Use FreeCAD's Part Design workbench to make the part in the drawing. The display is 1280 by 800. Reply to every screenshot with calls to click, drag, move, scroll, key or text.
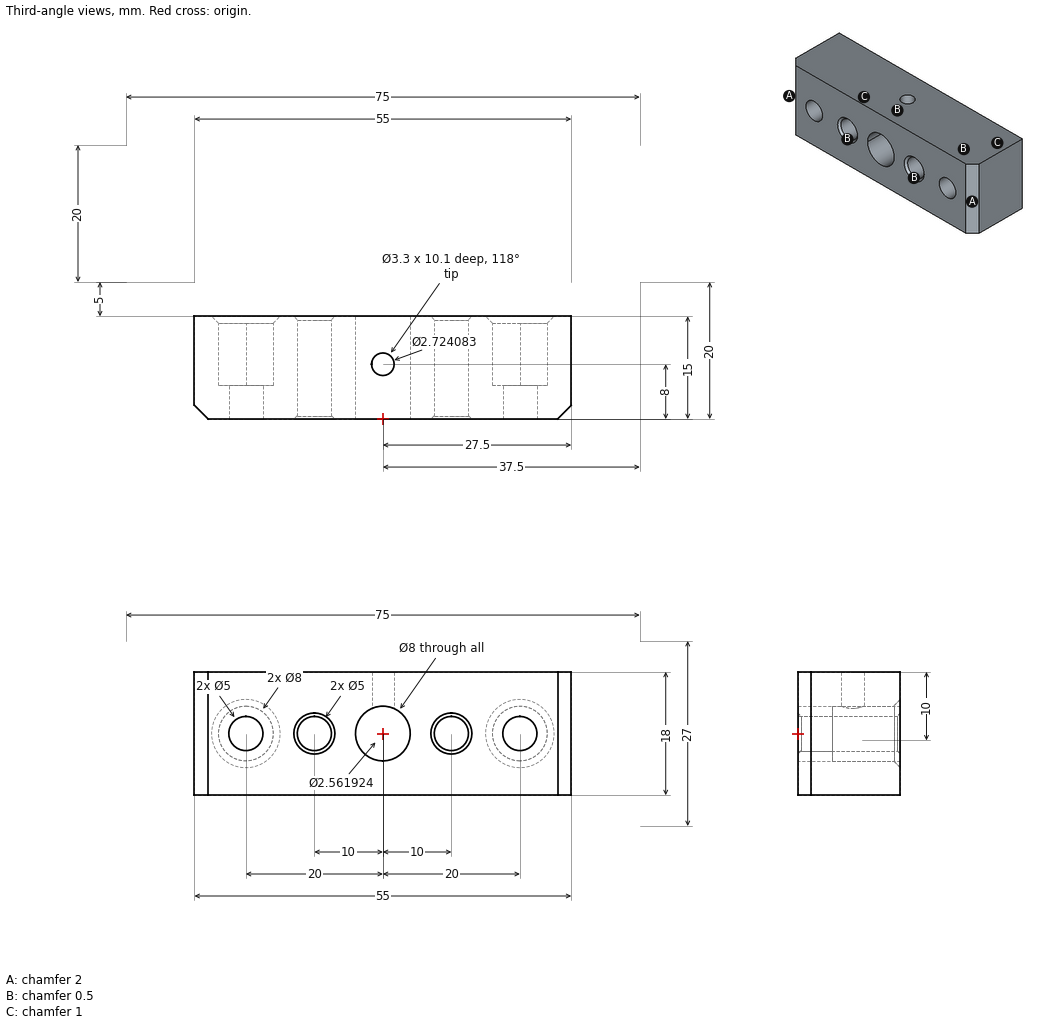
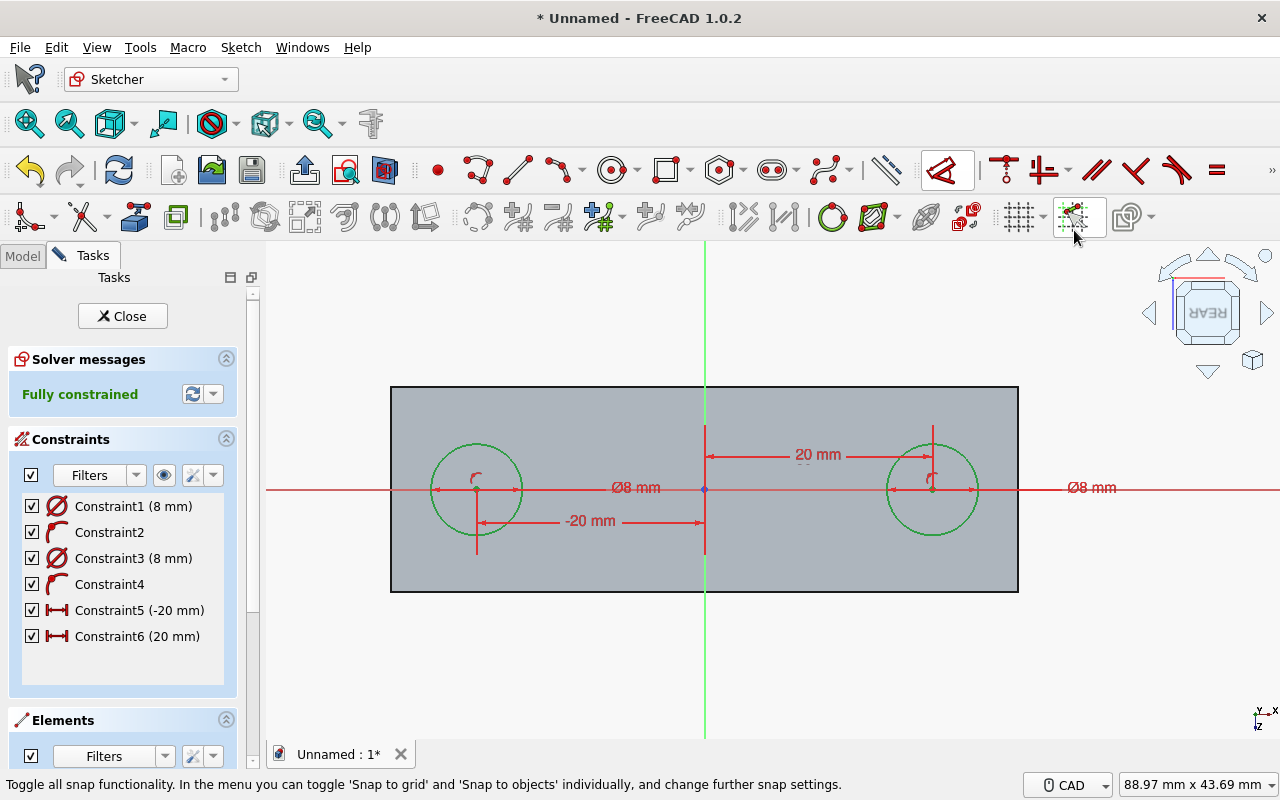
click(123, 316)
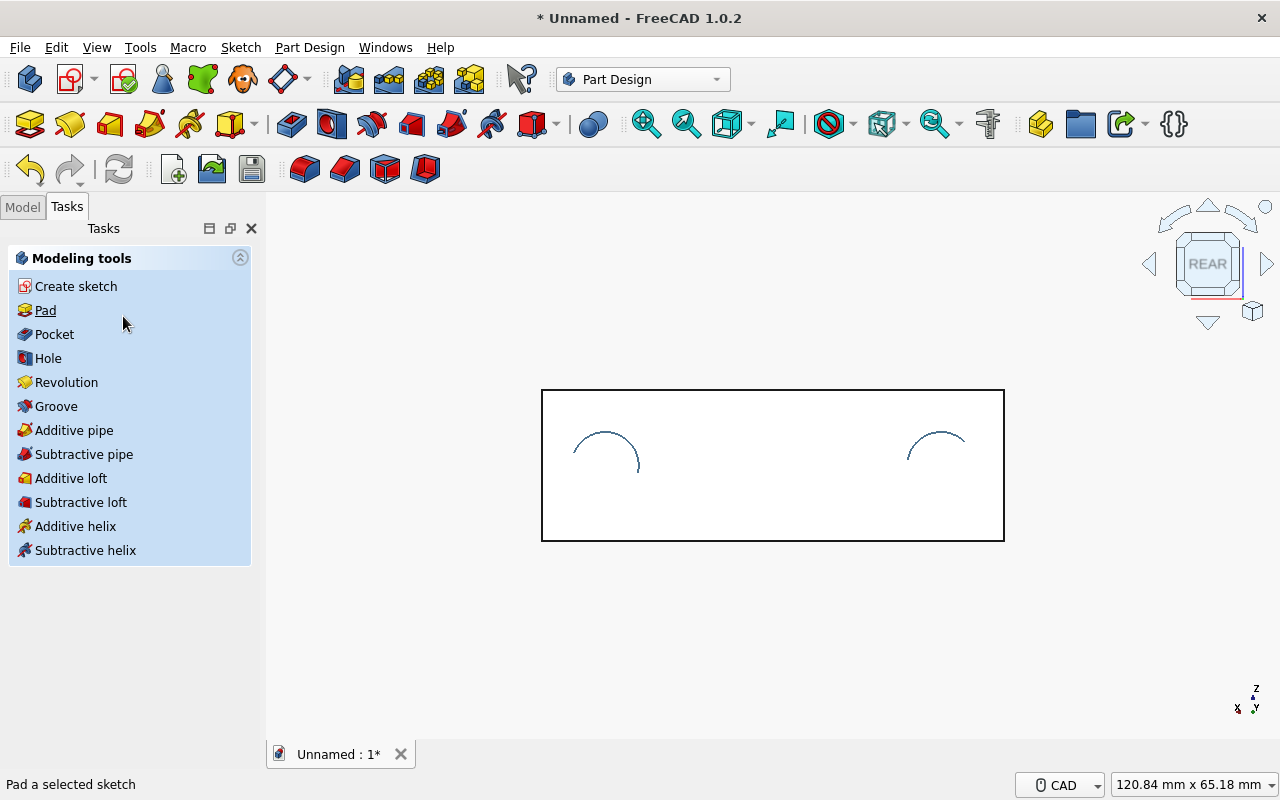
click(292, 124)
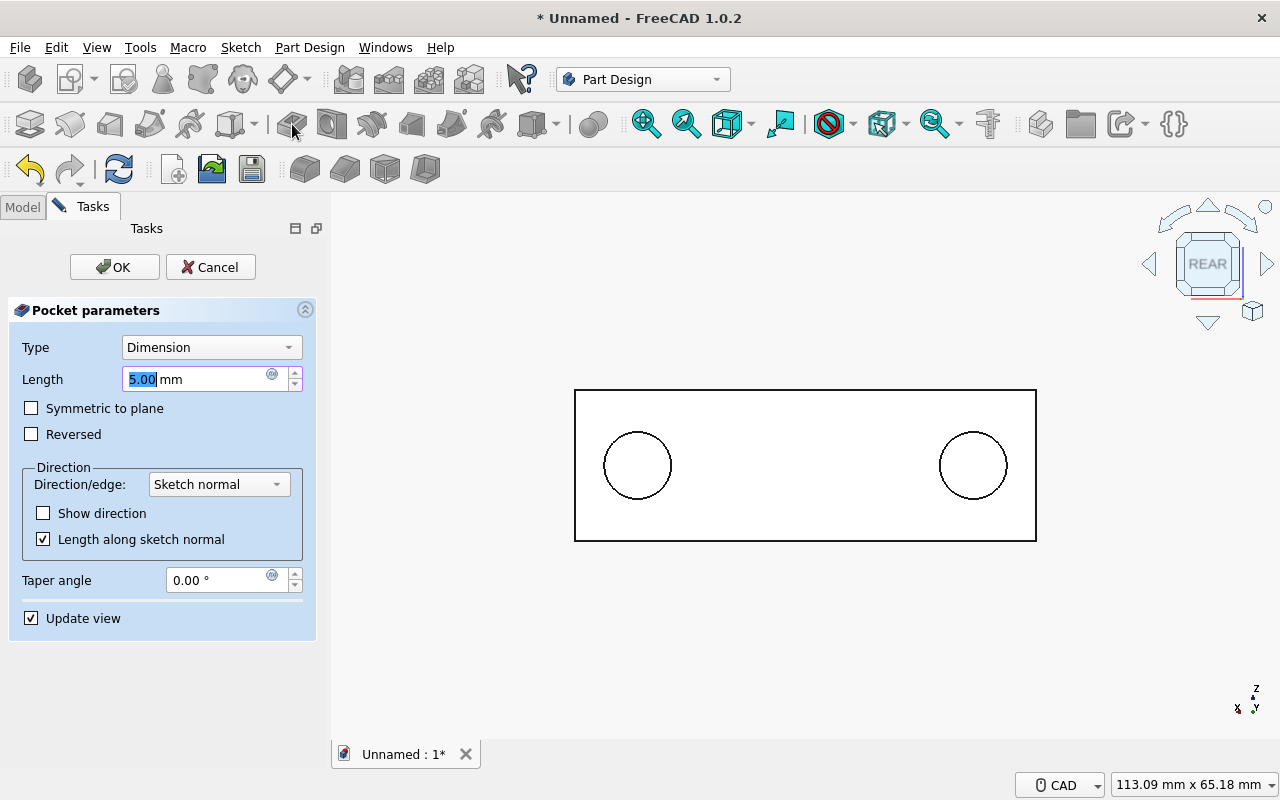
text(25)
key(Tab)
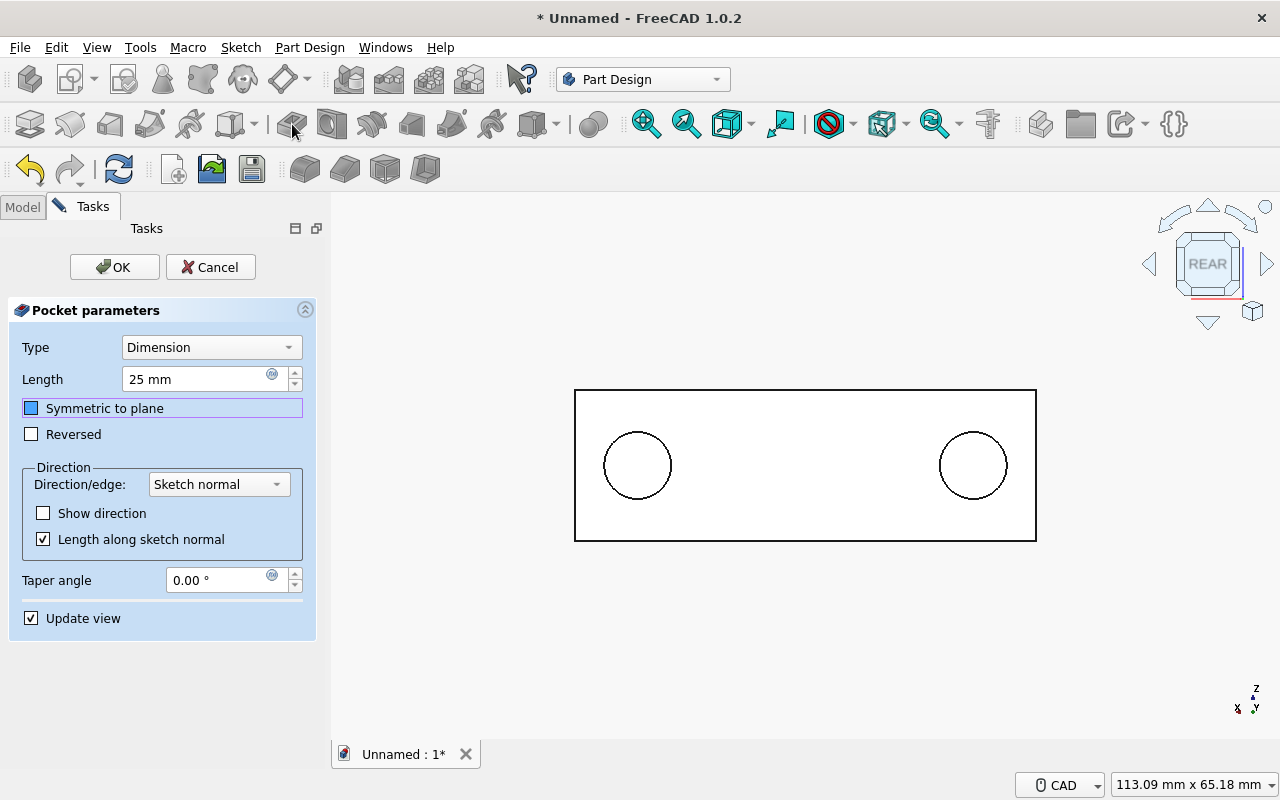
click(115, 267)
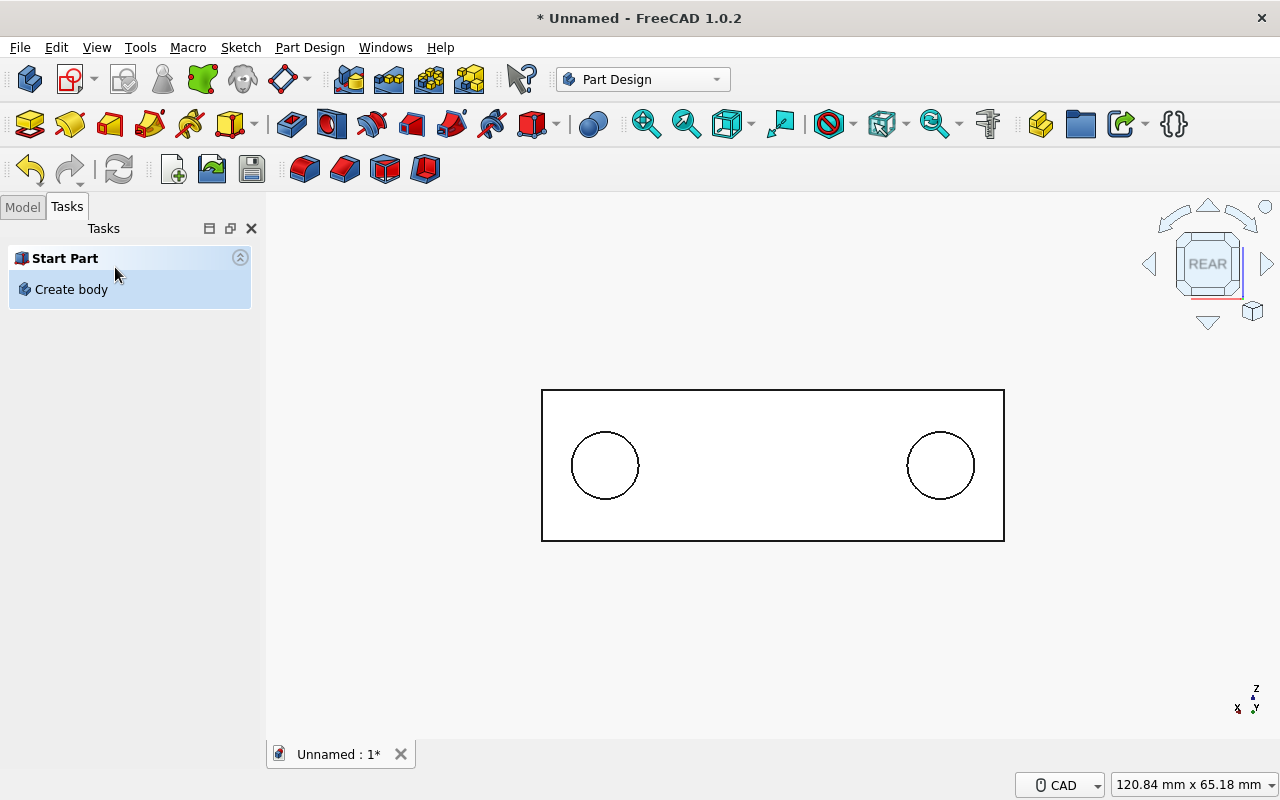
click(773, 465)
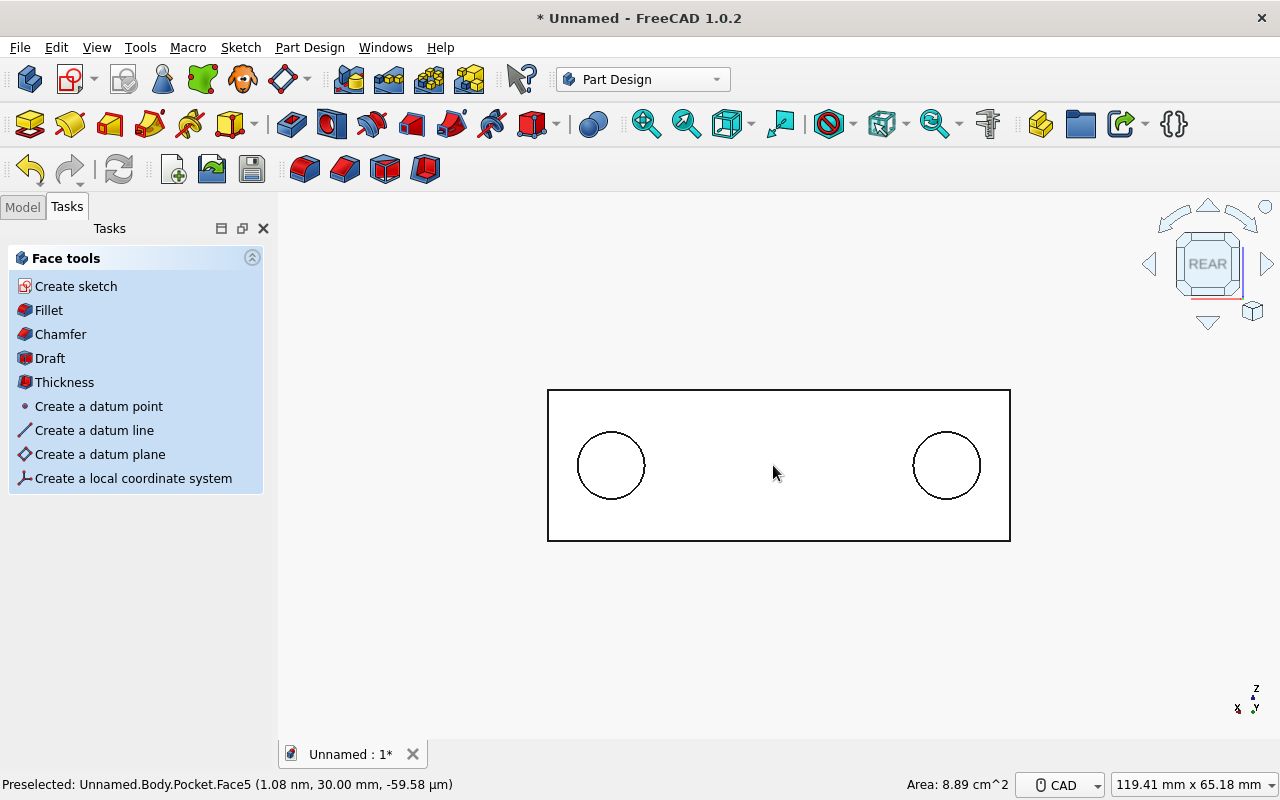
click(70, 80)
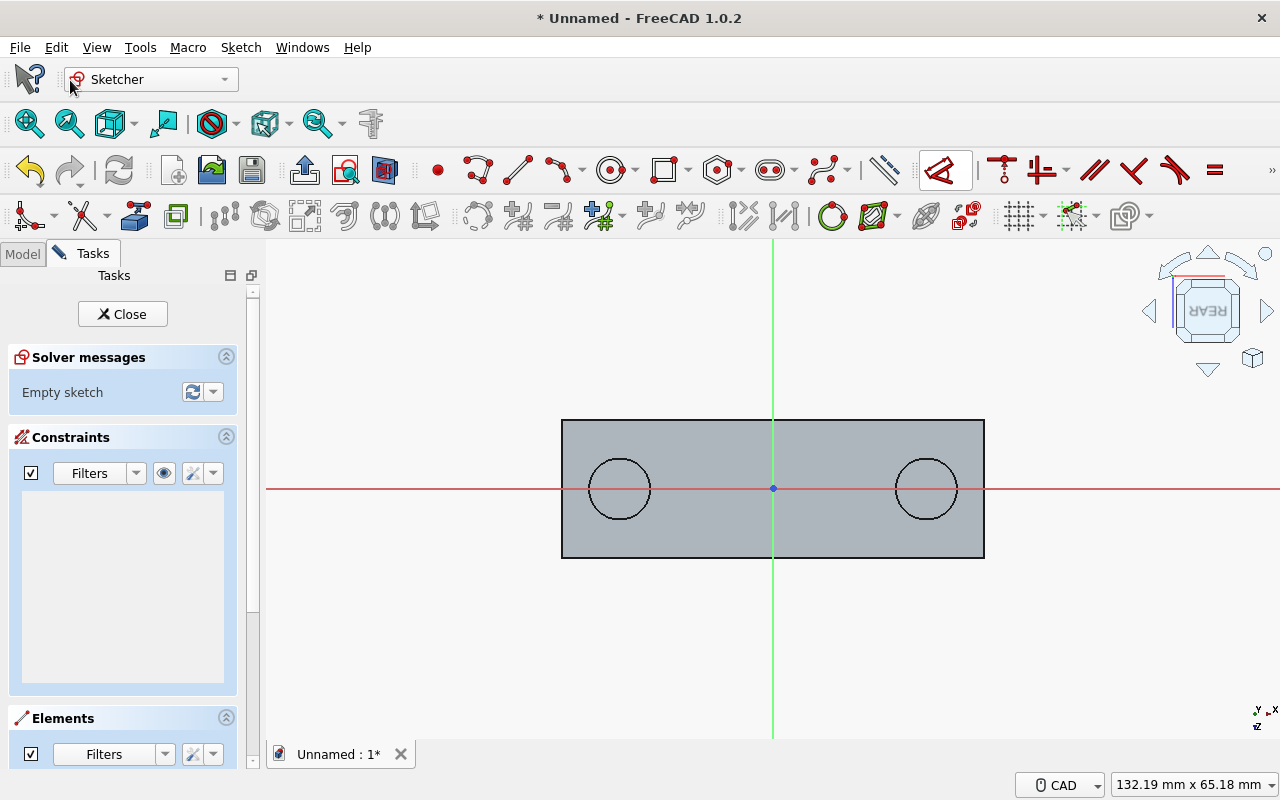
scroll(856, 489, up, 3)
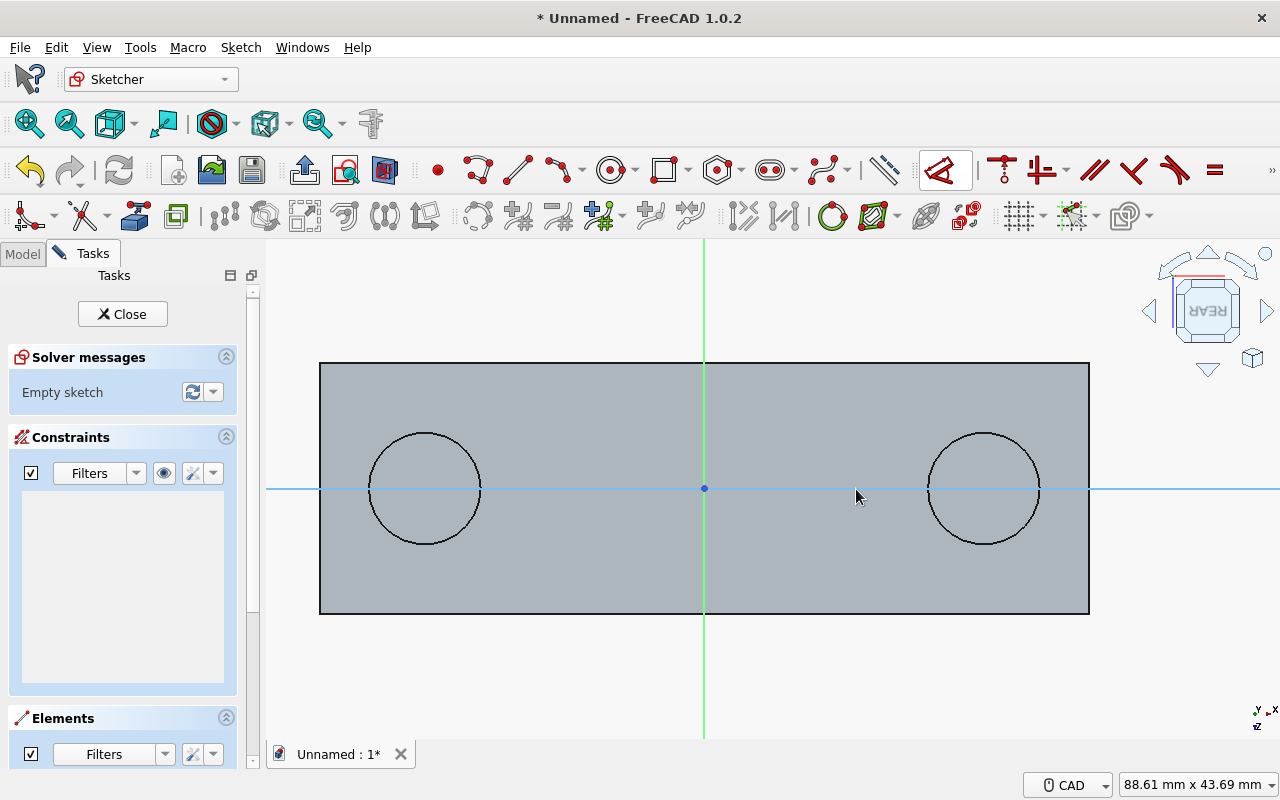
click(612, 170)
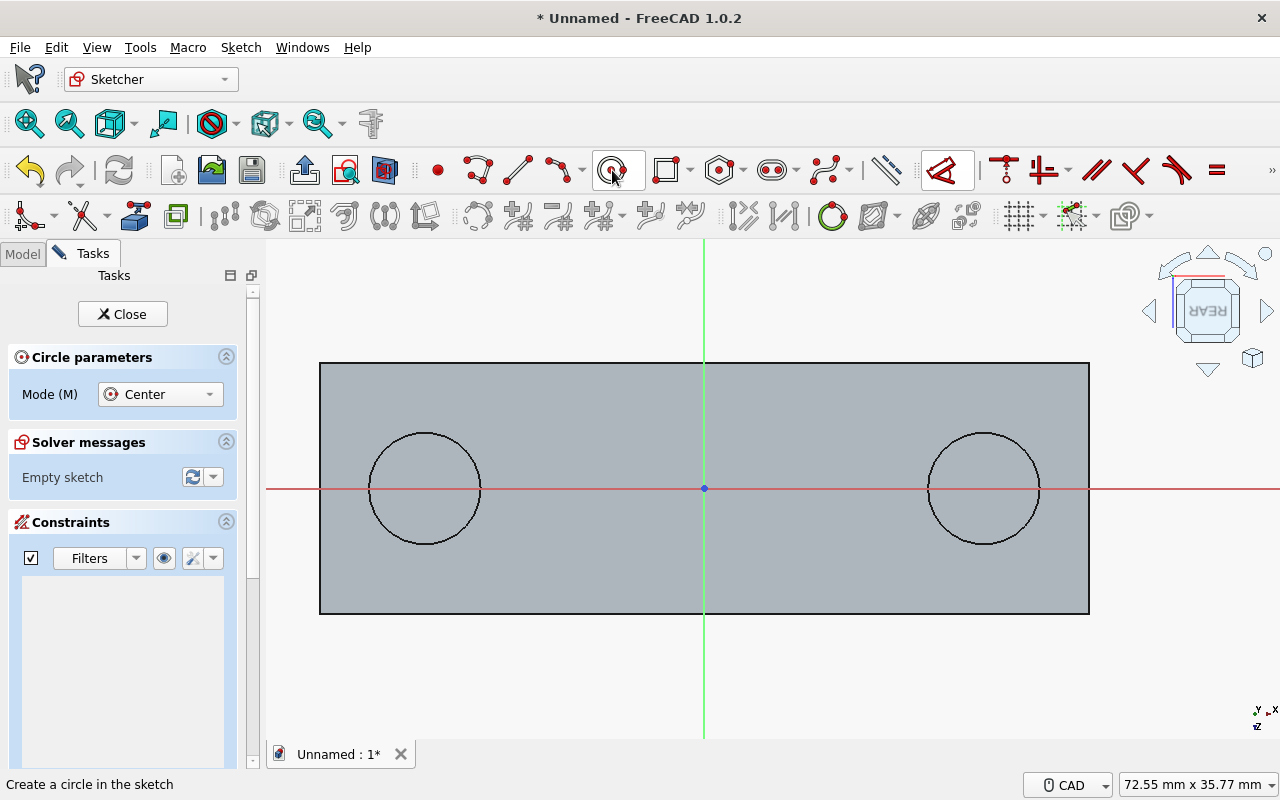
click(425, 489)
move(449, 464)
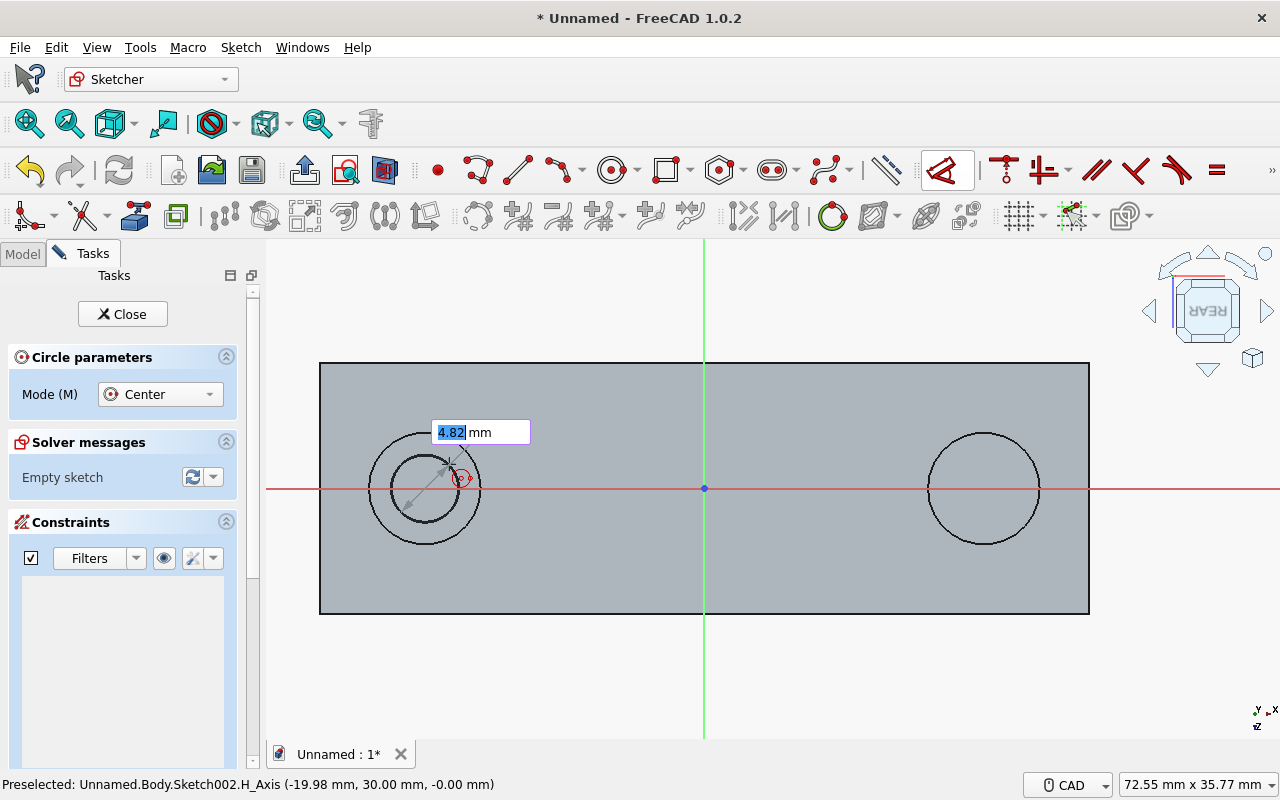
text(5)
key(Return)